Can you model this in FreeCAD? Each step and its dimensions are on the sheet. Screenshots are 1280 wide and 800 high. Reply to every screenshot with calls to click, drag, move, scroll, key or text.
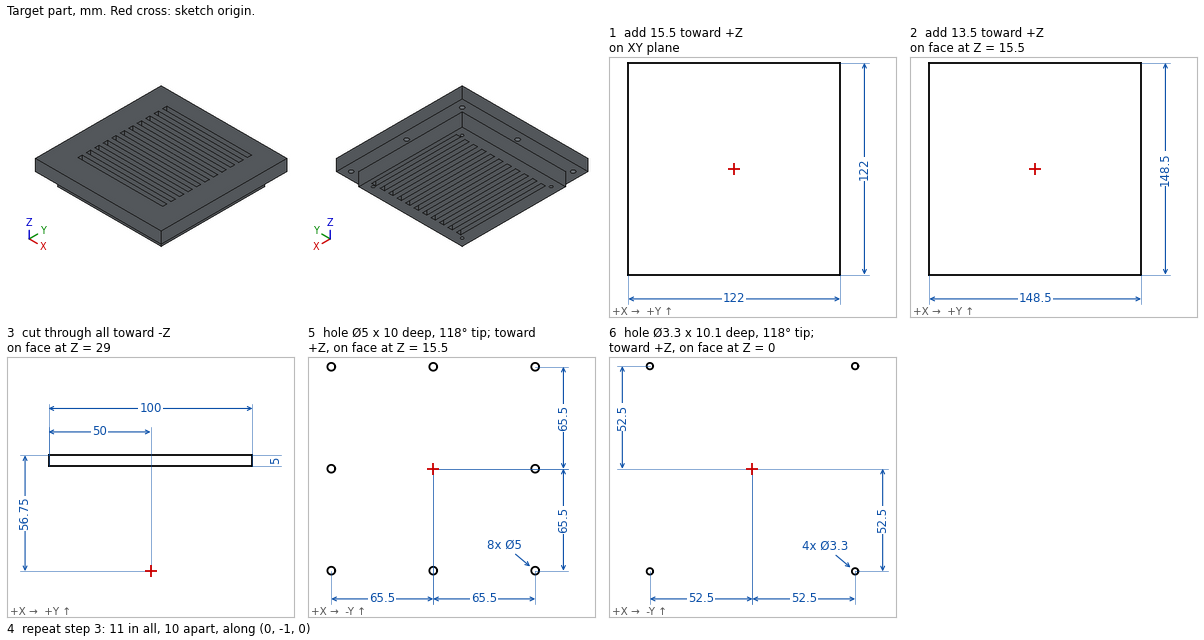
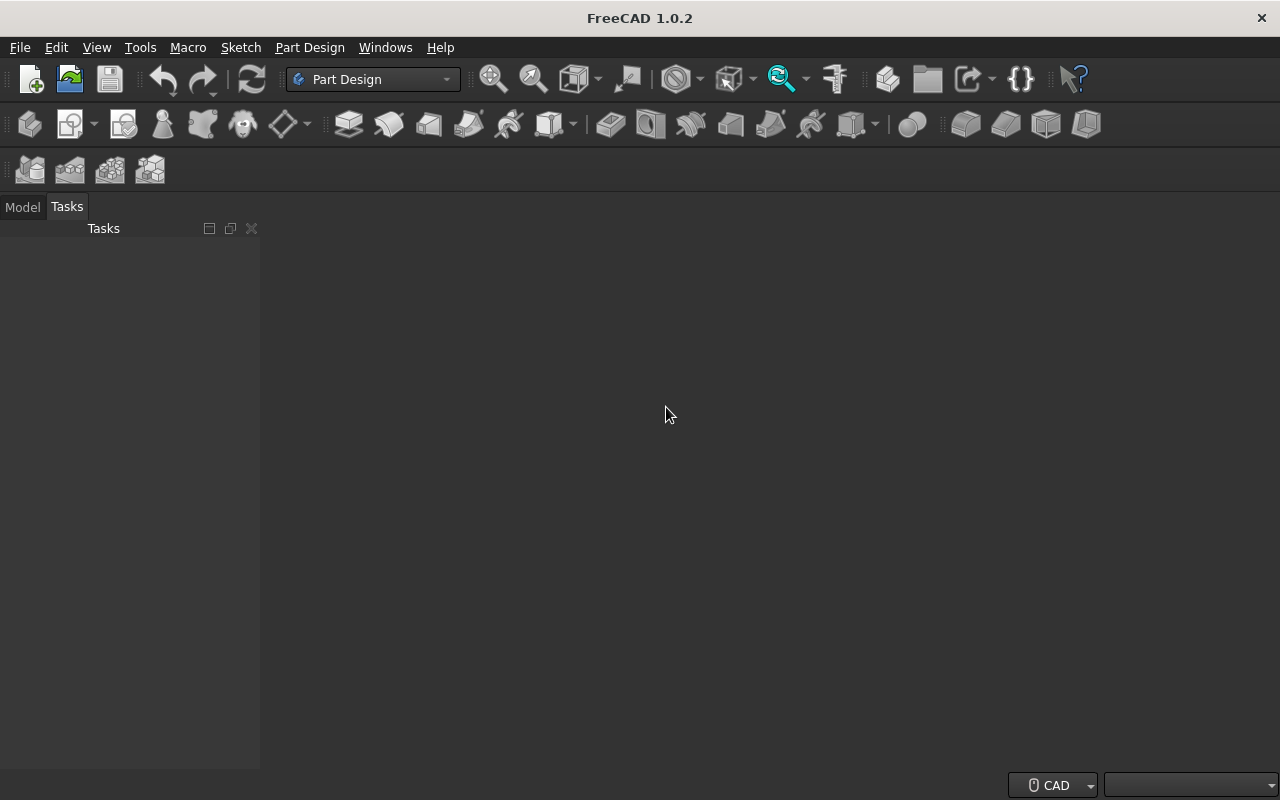
click(30, 80)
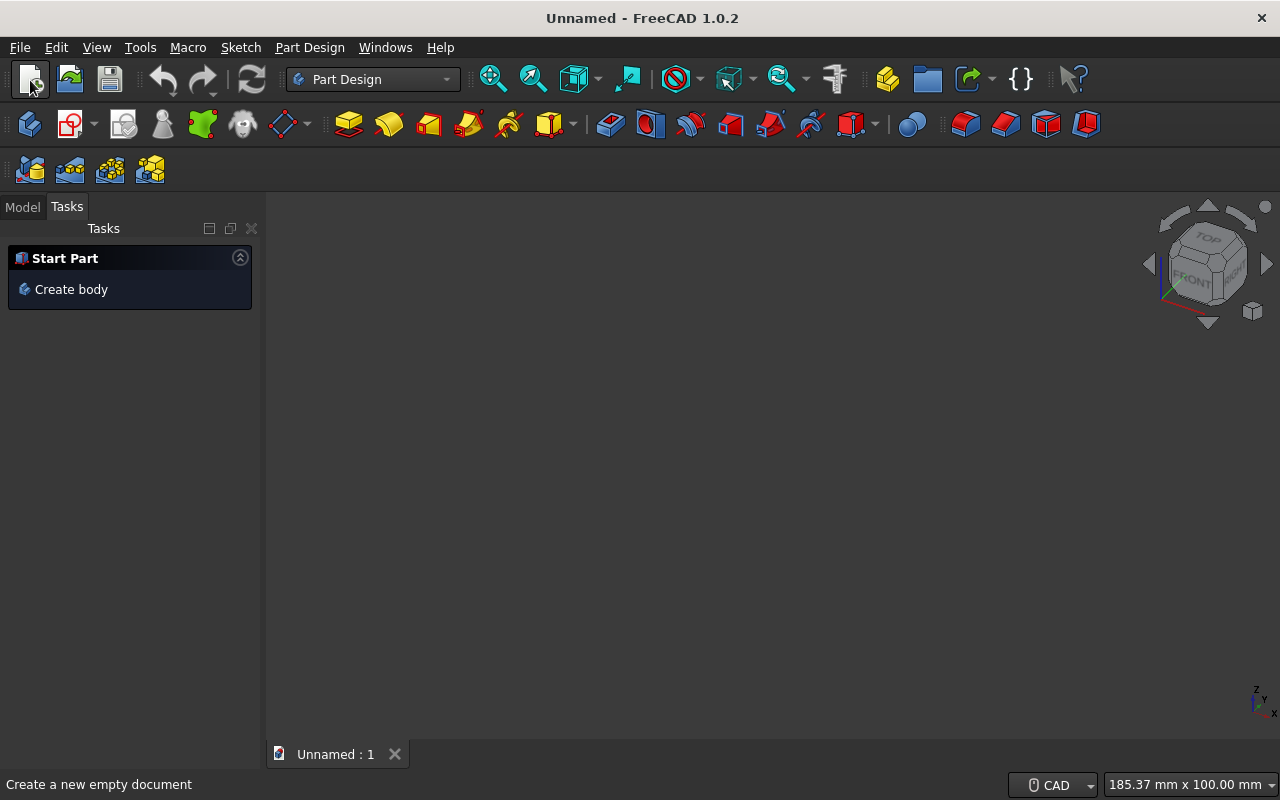
click(70, 124)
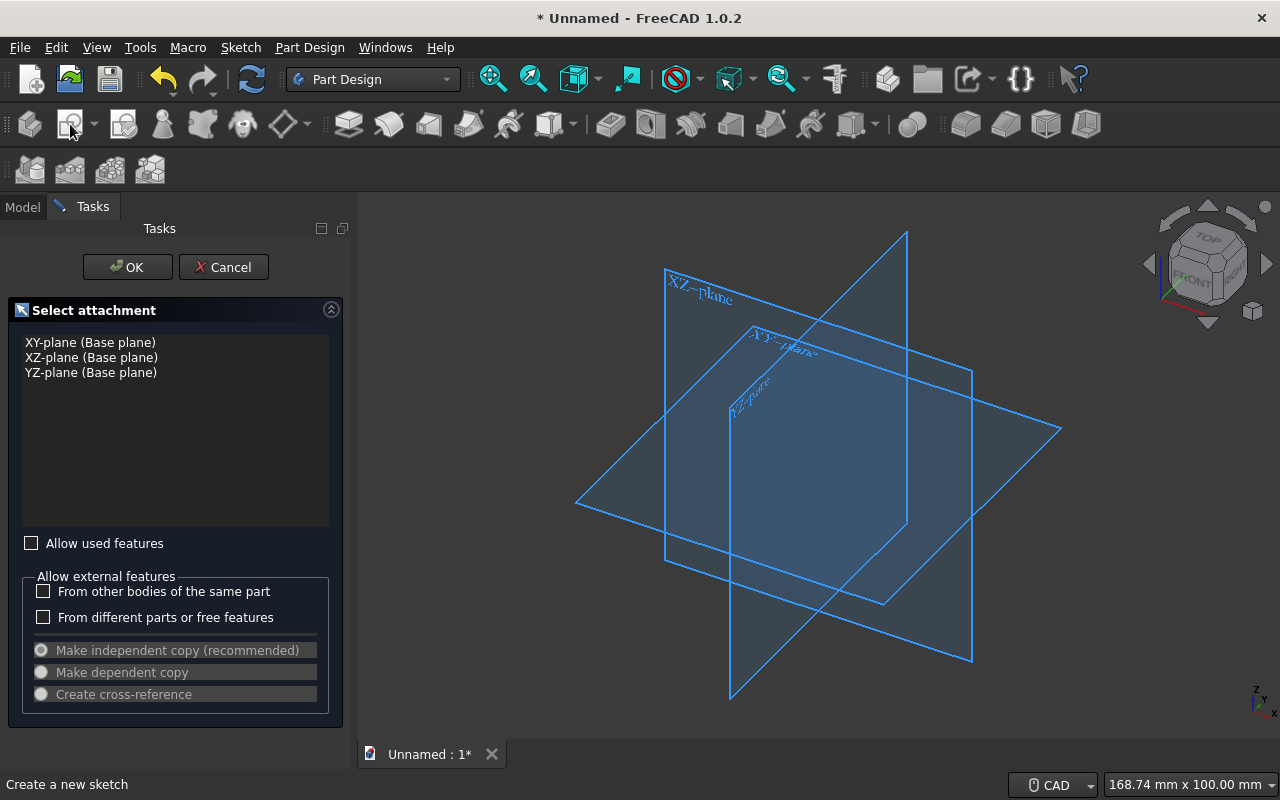
click(82, 342)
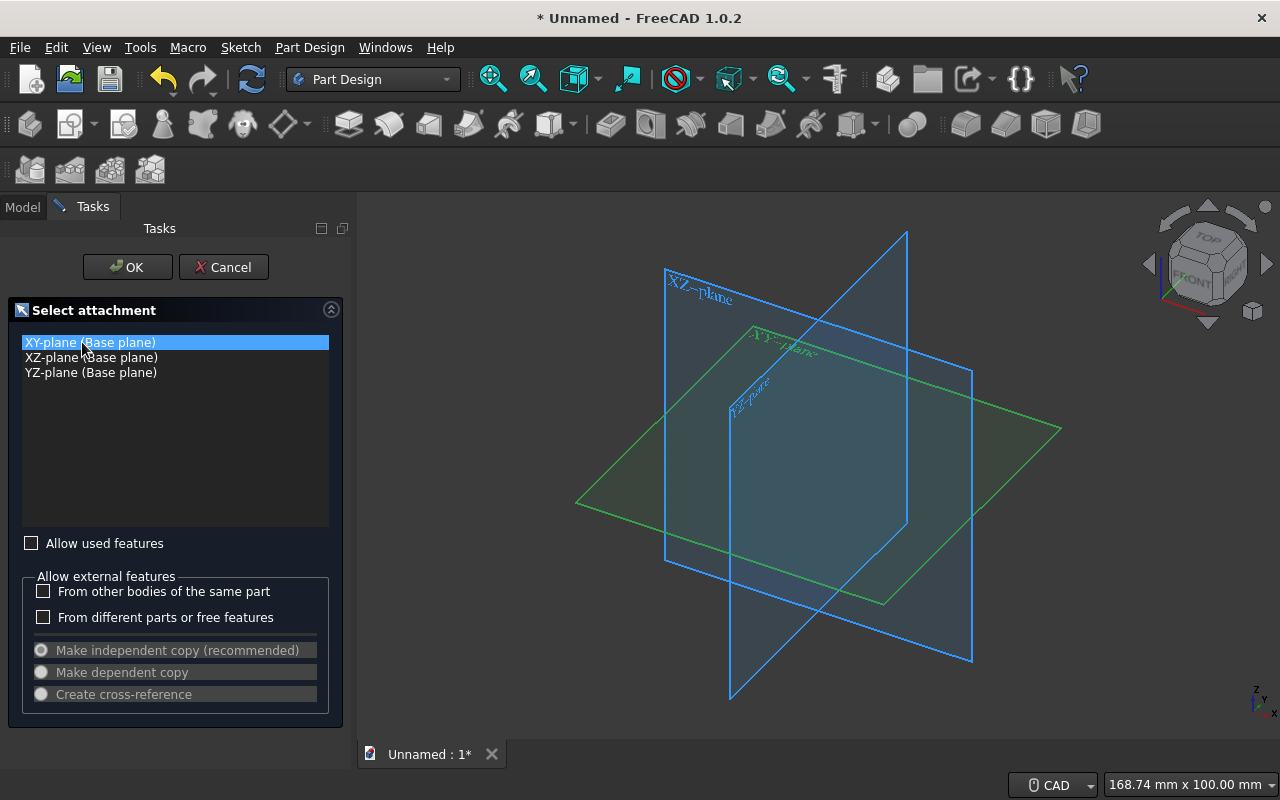
click(128, 267)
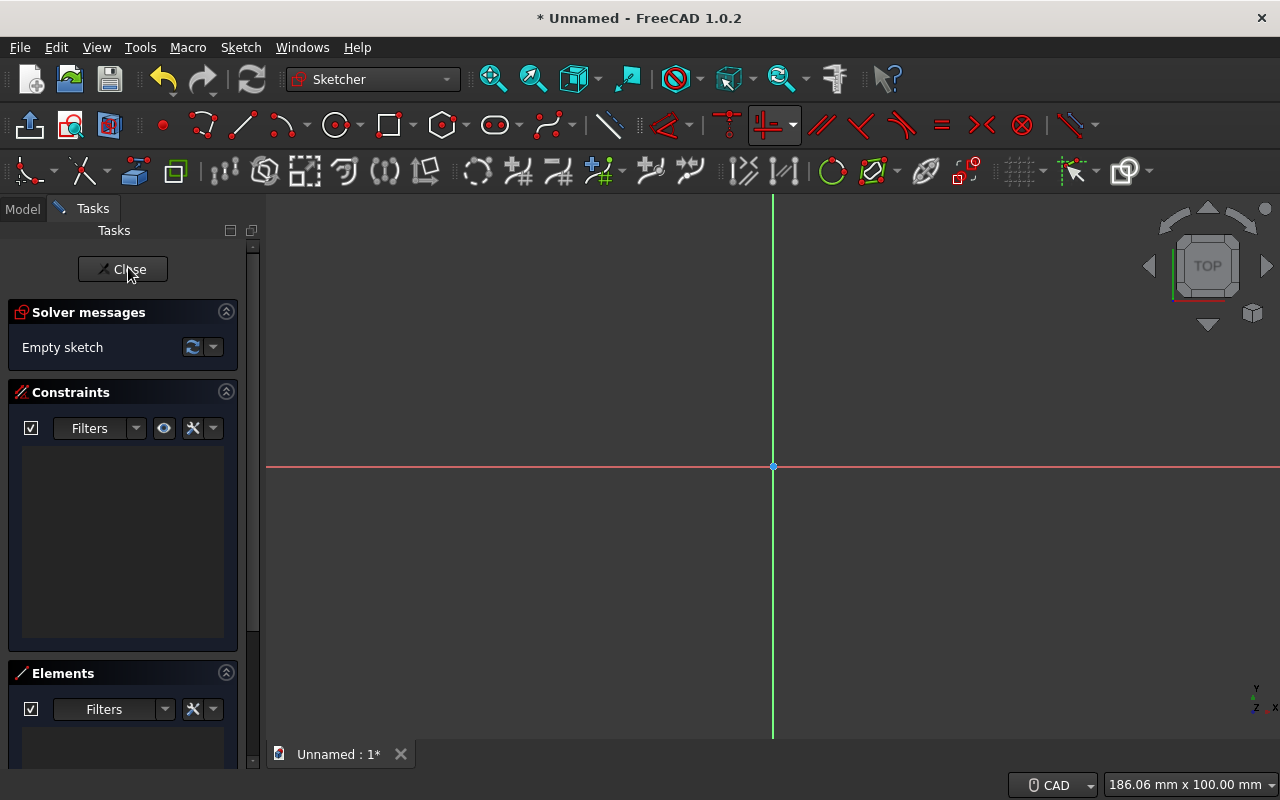
scroll(621, 466, down, 3)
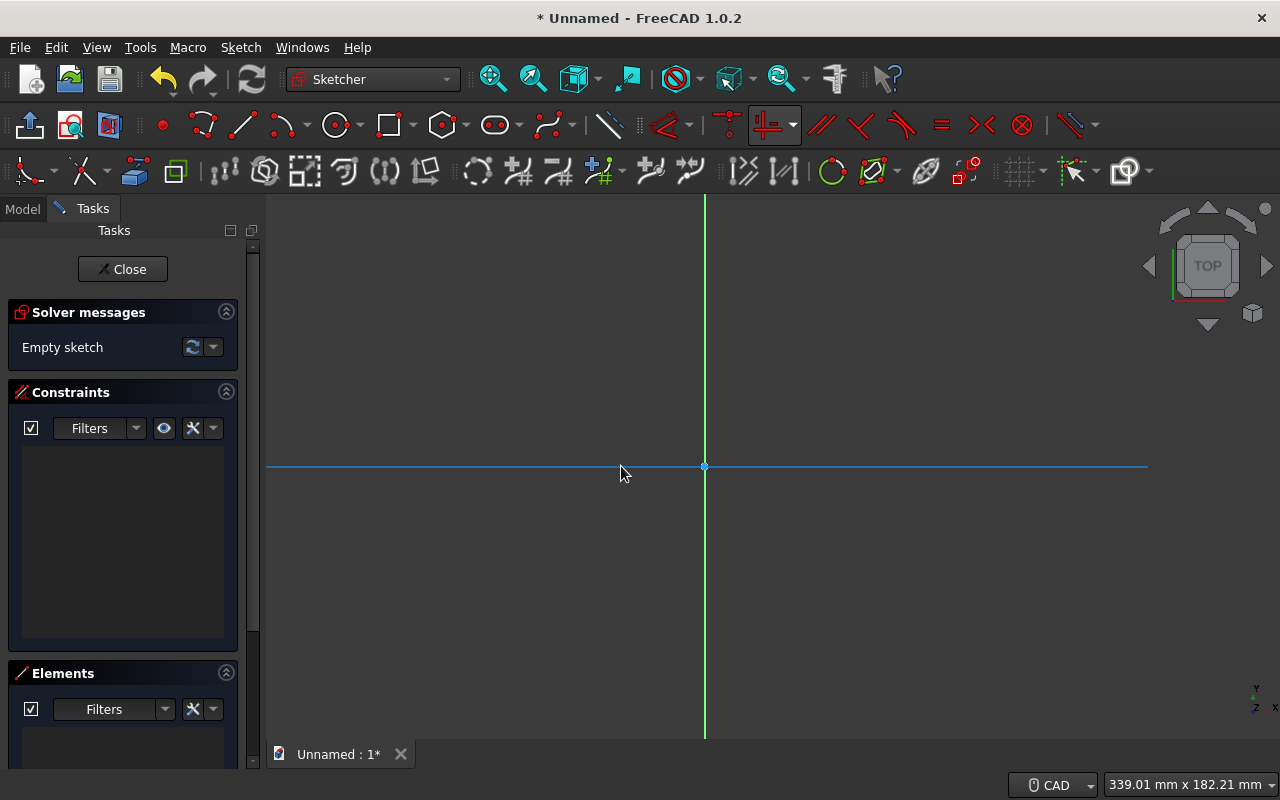
click(416, 126)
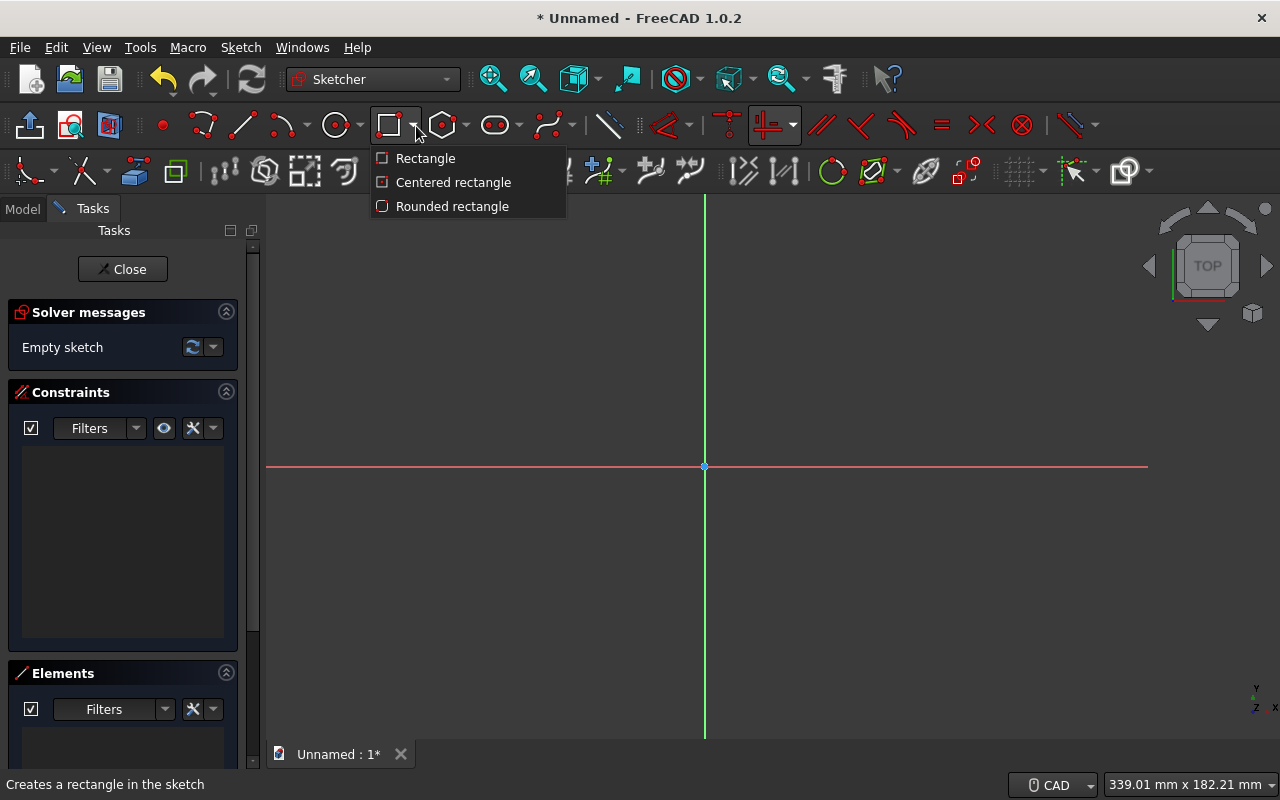
click(468, 182)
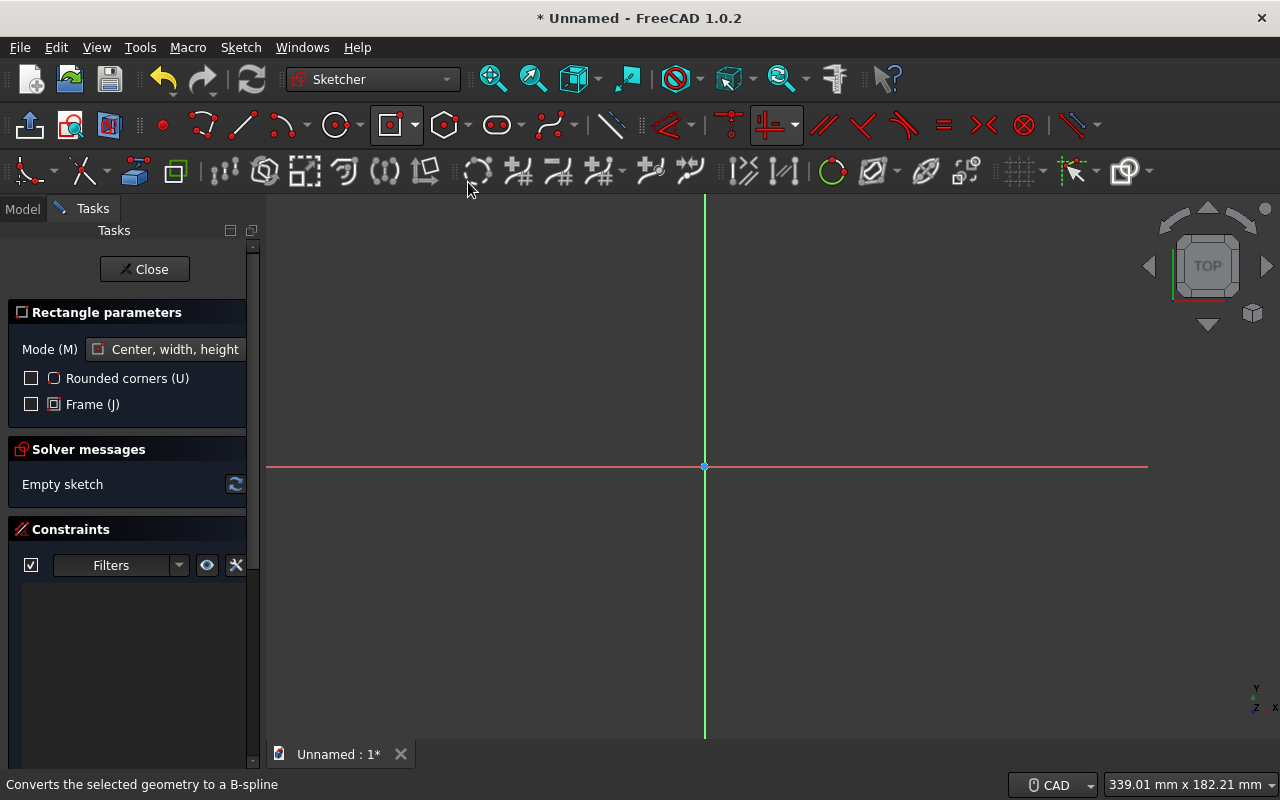
click(705, 466)
move(887, 284)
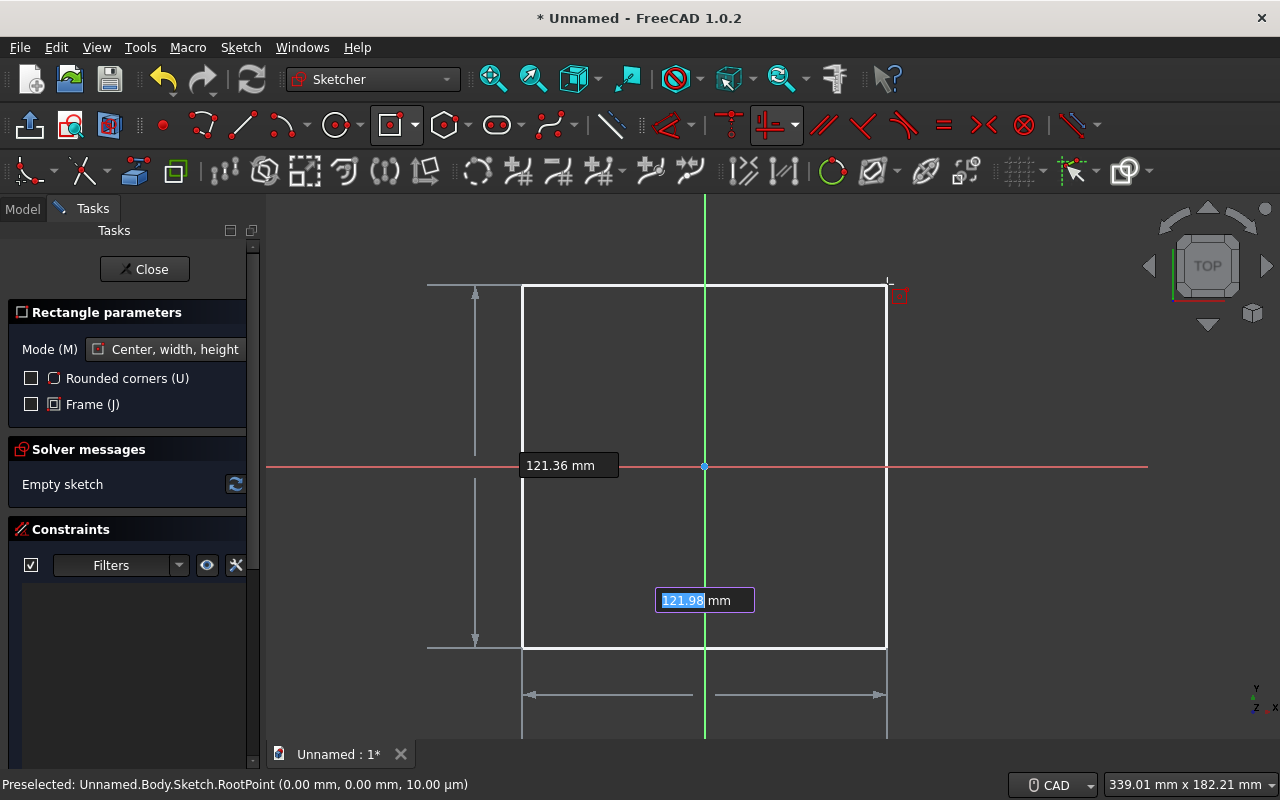
text(122)
key(Tab)
text(122)
key(Return)
key(Escape)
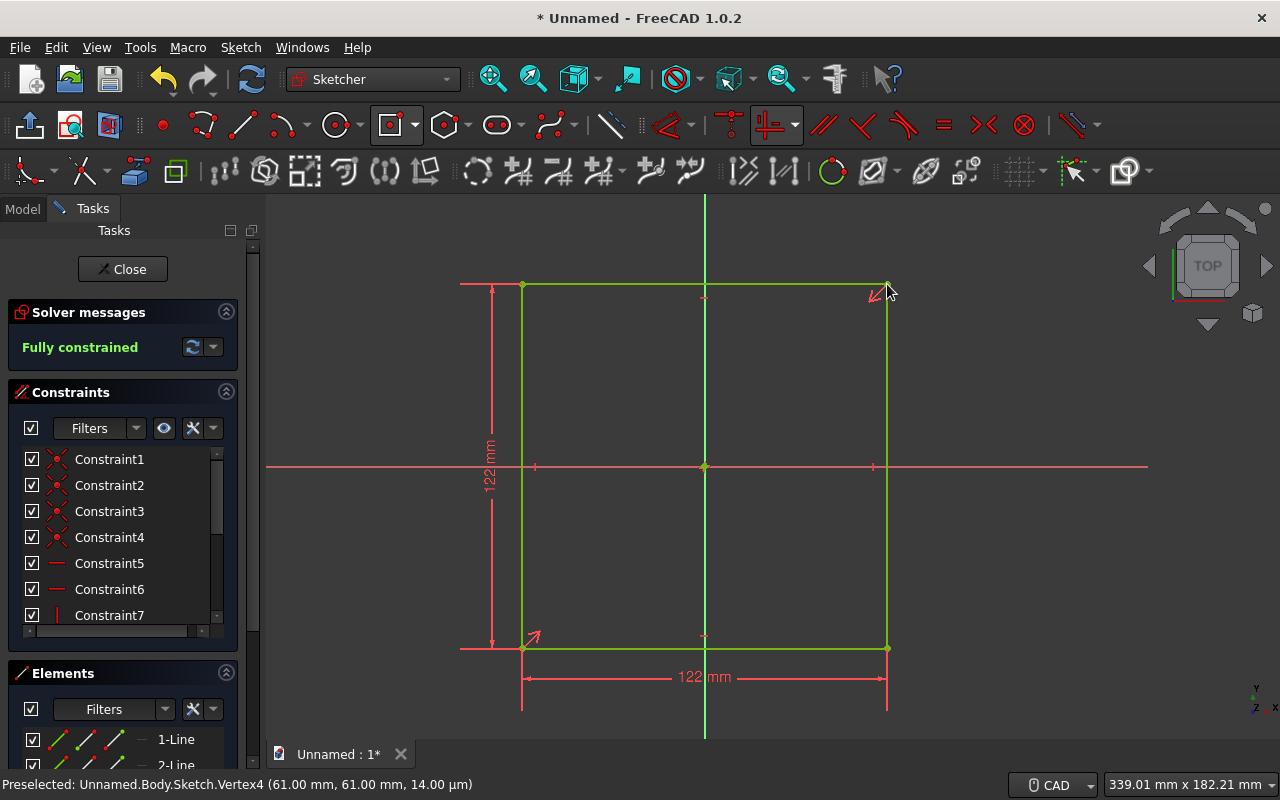
click(123, 269)